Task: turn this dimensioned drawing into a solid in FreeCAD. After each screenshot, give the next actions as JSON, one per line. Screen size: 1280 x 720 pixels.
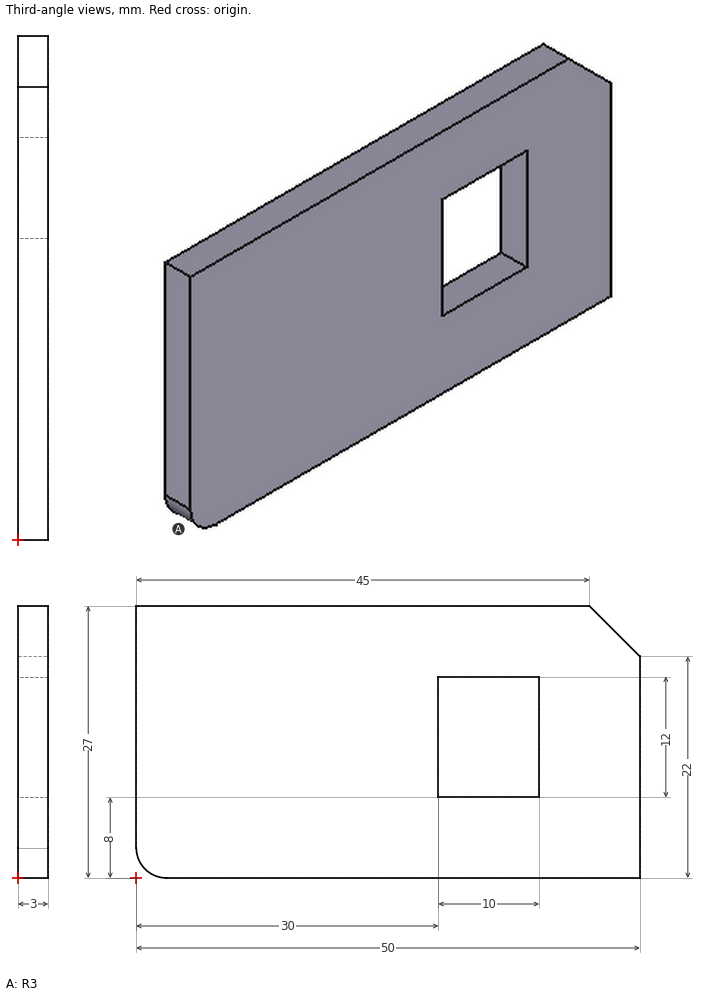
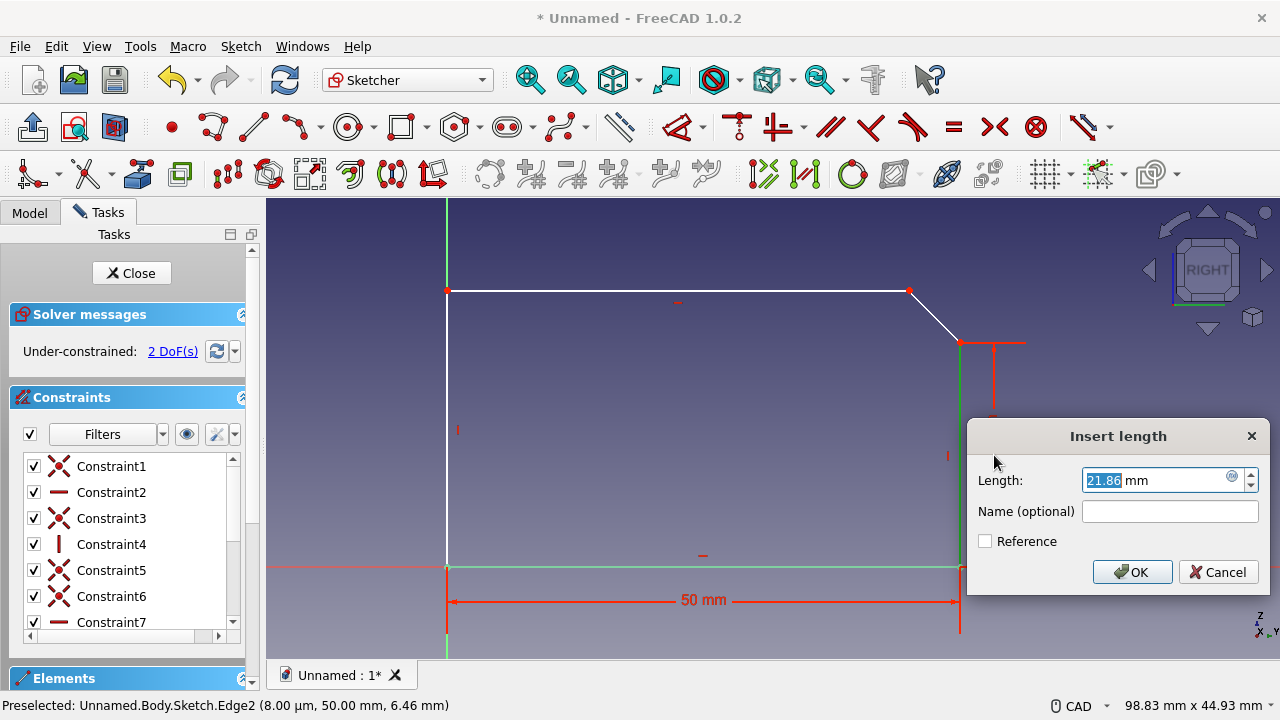
{"action": "type", "text": "22"}
{"action": "key", "text": "Return"}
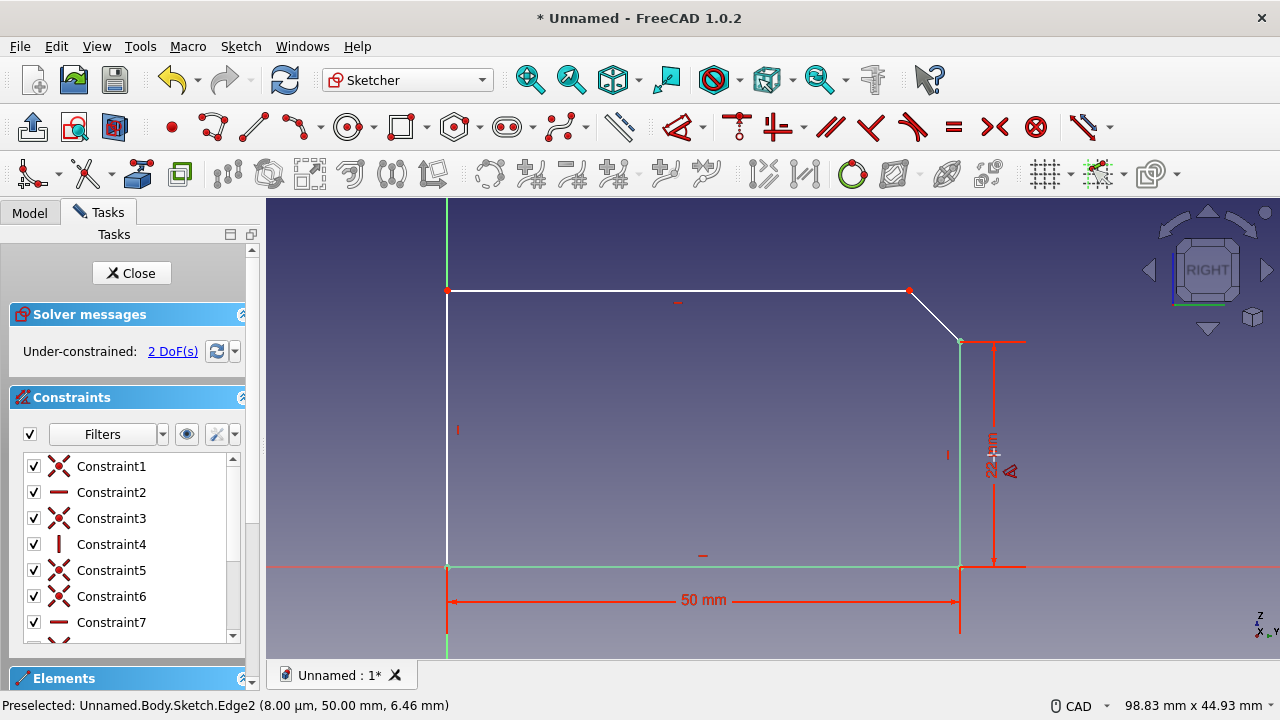
{"action": "left_click", "coordinate": [770, 291]}
{"action": "left_click", "coordinate": [678, 257]}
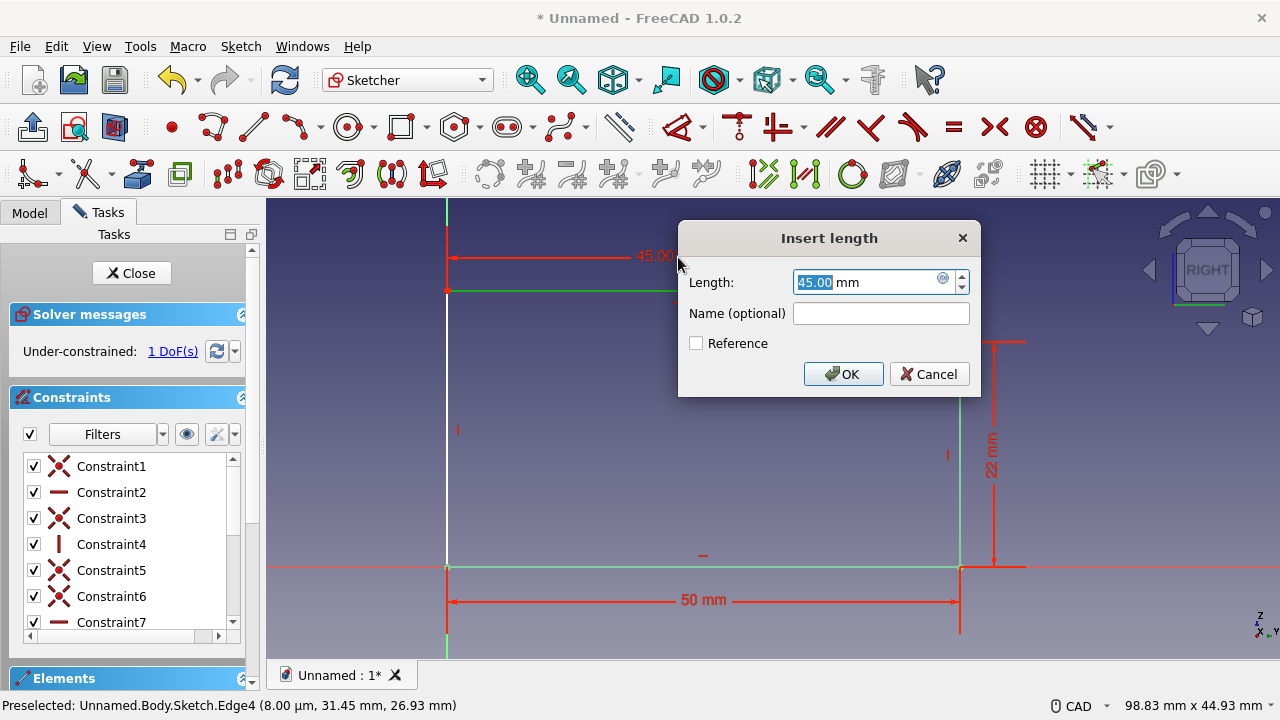
{"action": "type", "text": "45"}
{"action": "key", "text": "Return"}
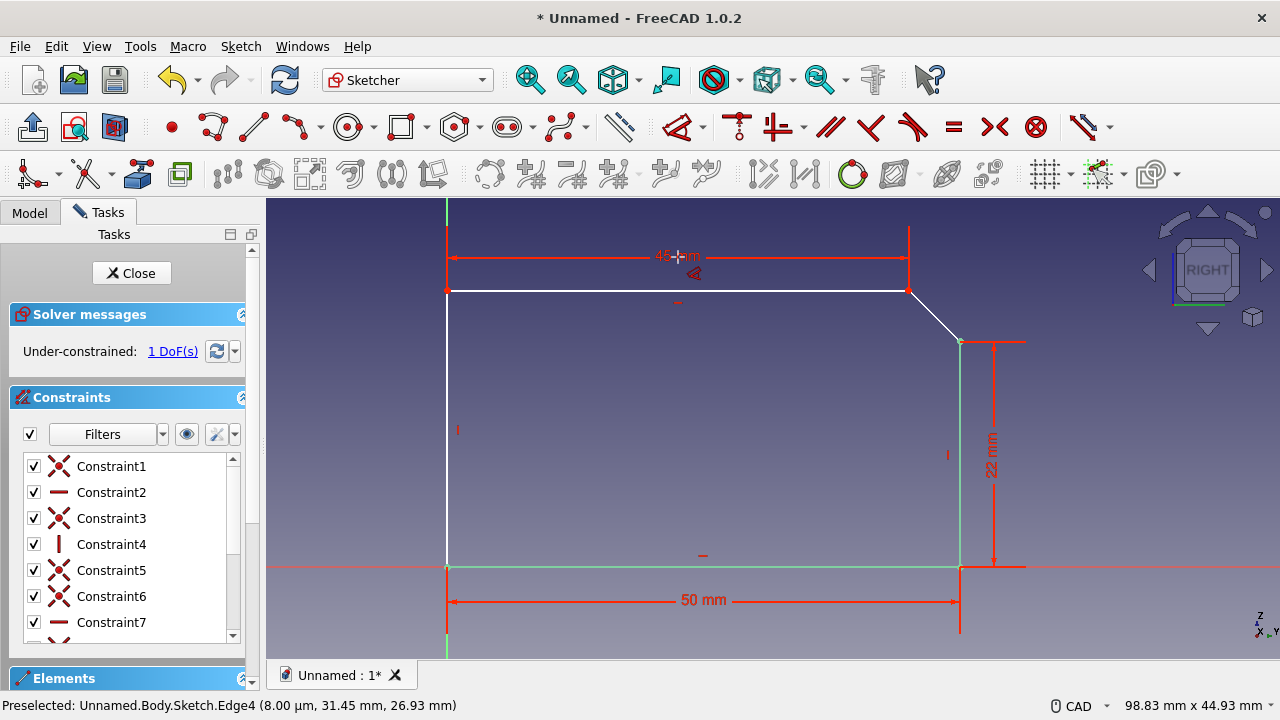
{"action": "left_click", "coordinate": [447, 374]}
{"action": "left_click", "coordinate": [413, 429]}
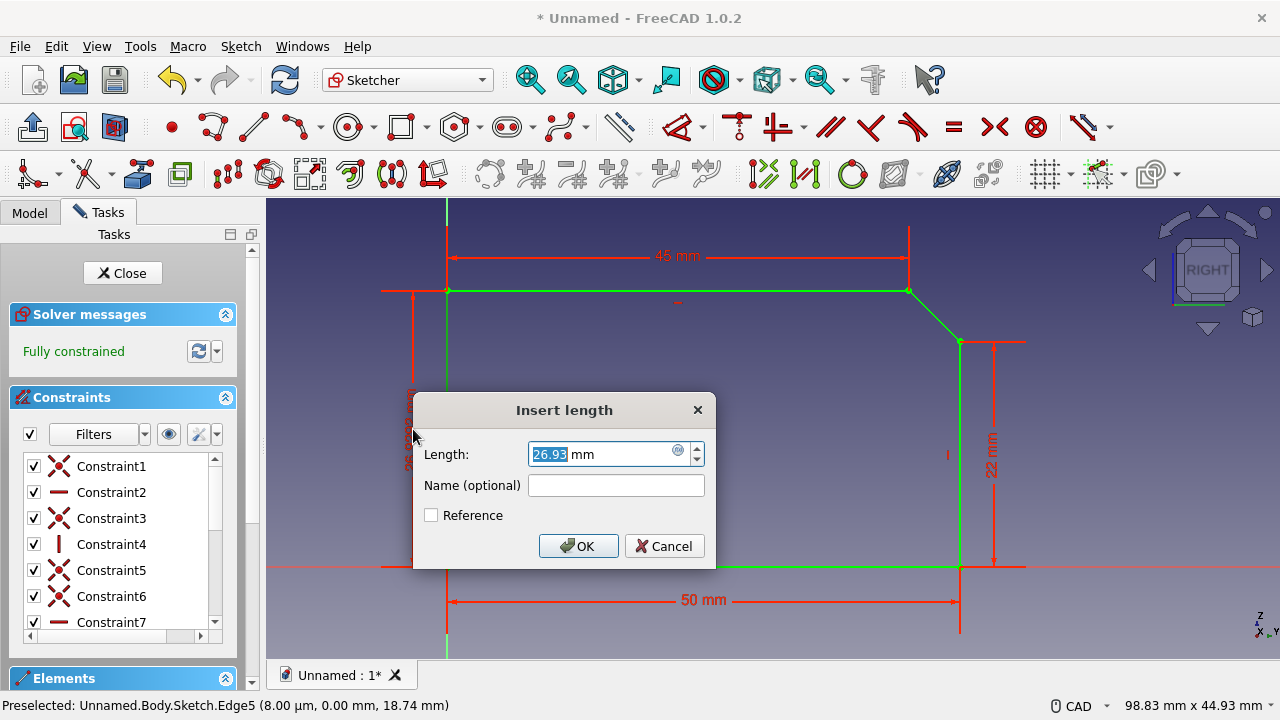
{"action": "type", "text": "27"}
{"action": "key", "text": "Return"}
{"action": "key", "text": "Escape"}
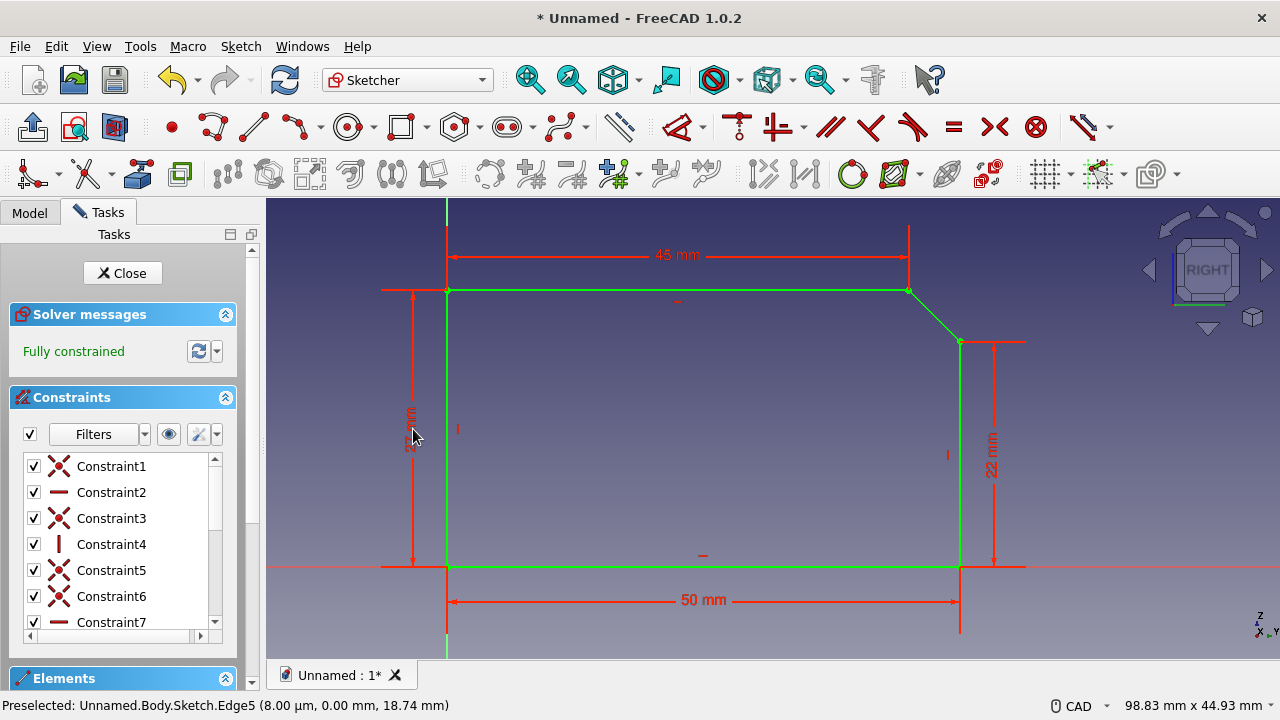
{"action": "left_click", "coordinate": [123, 273]}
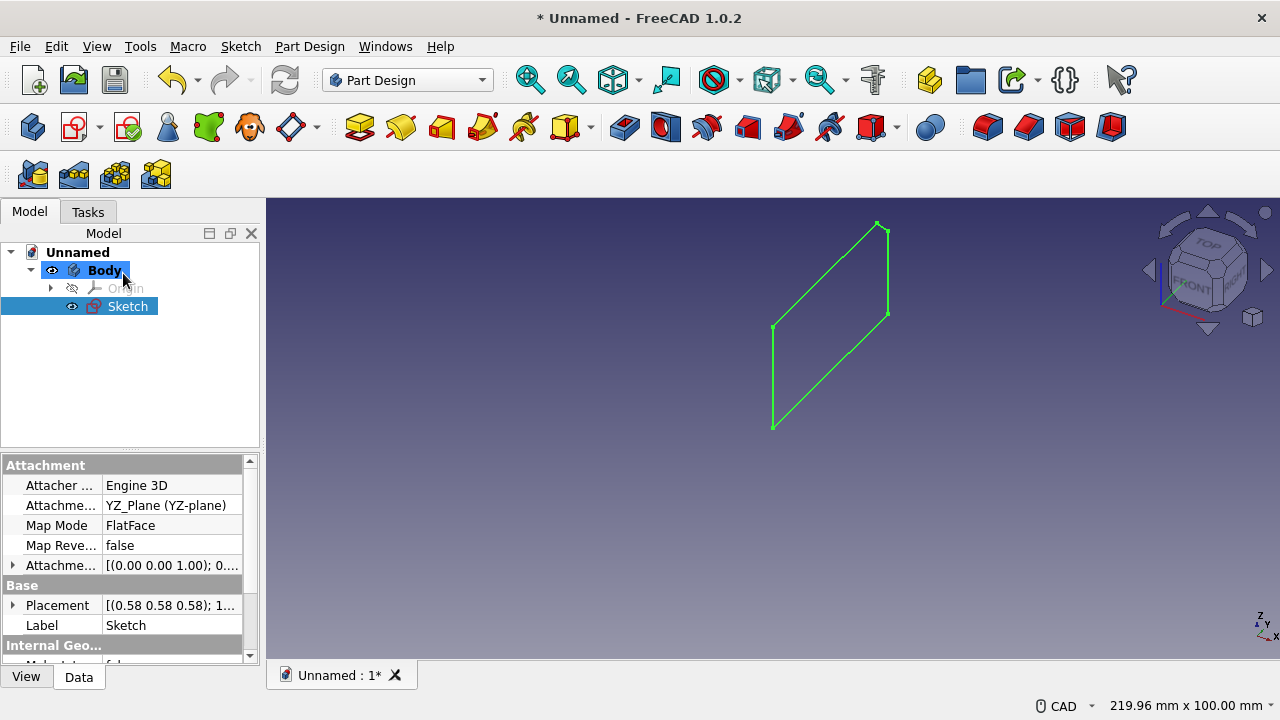
{"action": "left_click", "coordinate": [360, 128]}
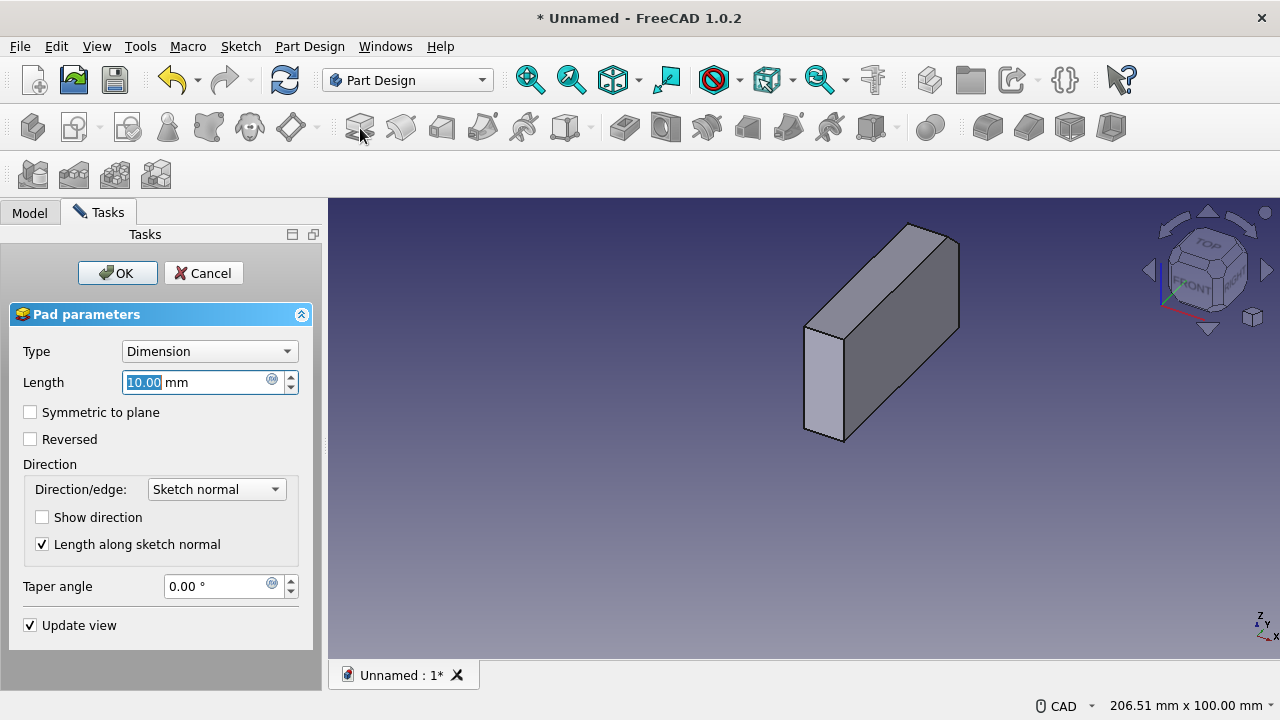
{"action": "type", "text": "3"}
{"action": "key", "text": "Tab"}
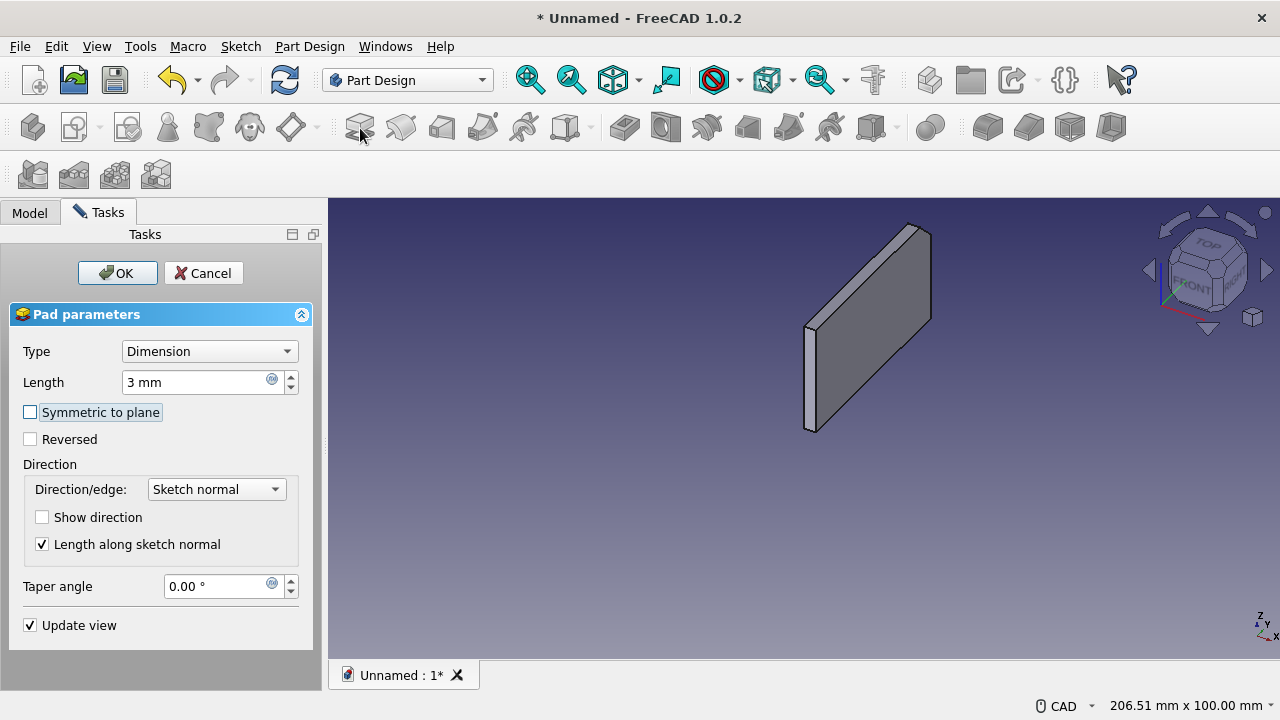
{"action": "left_click", "coordinate": [118, 273]}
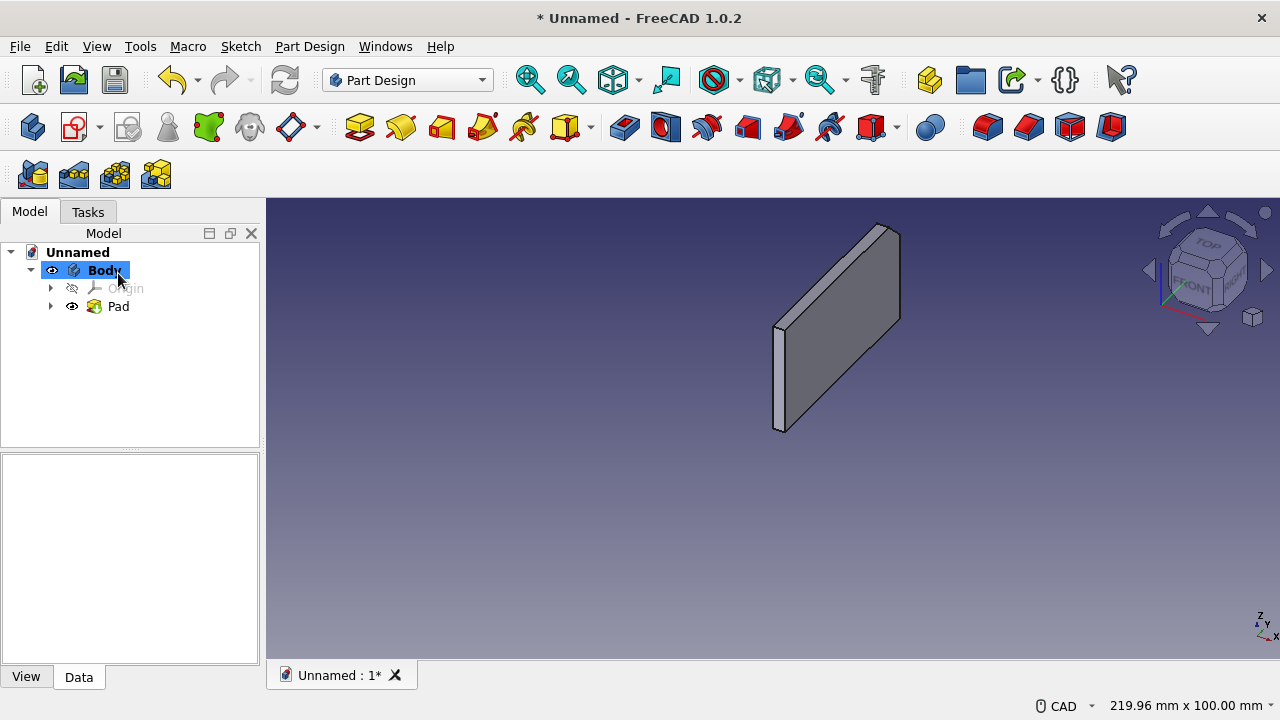
{"action": "scroll", "coordinate": [779, 429], "scroll_direction": "up", "scroll_amount": 6}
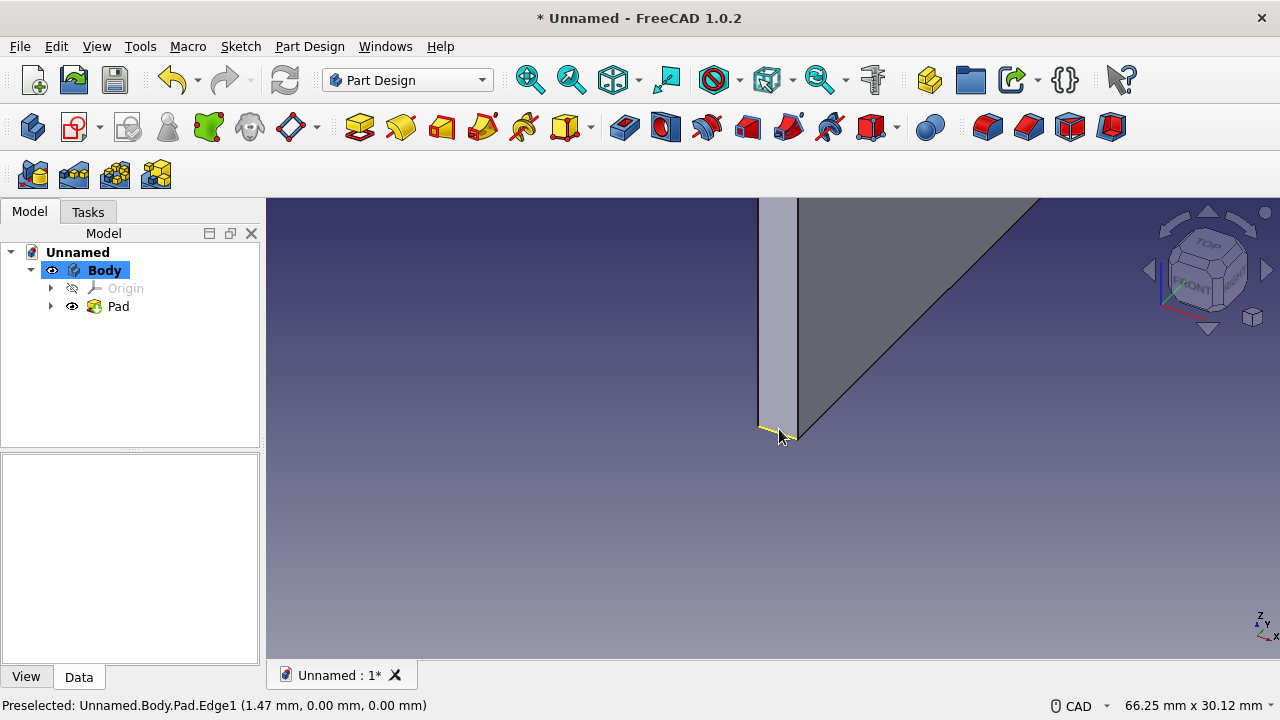
{"action": "left_click", "coordinate": [531, 80]}